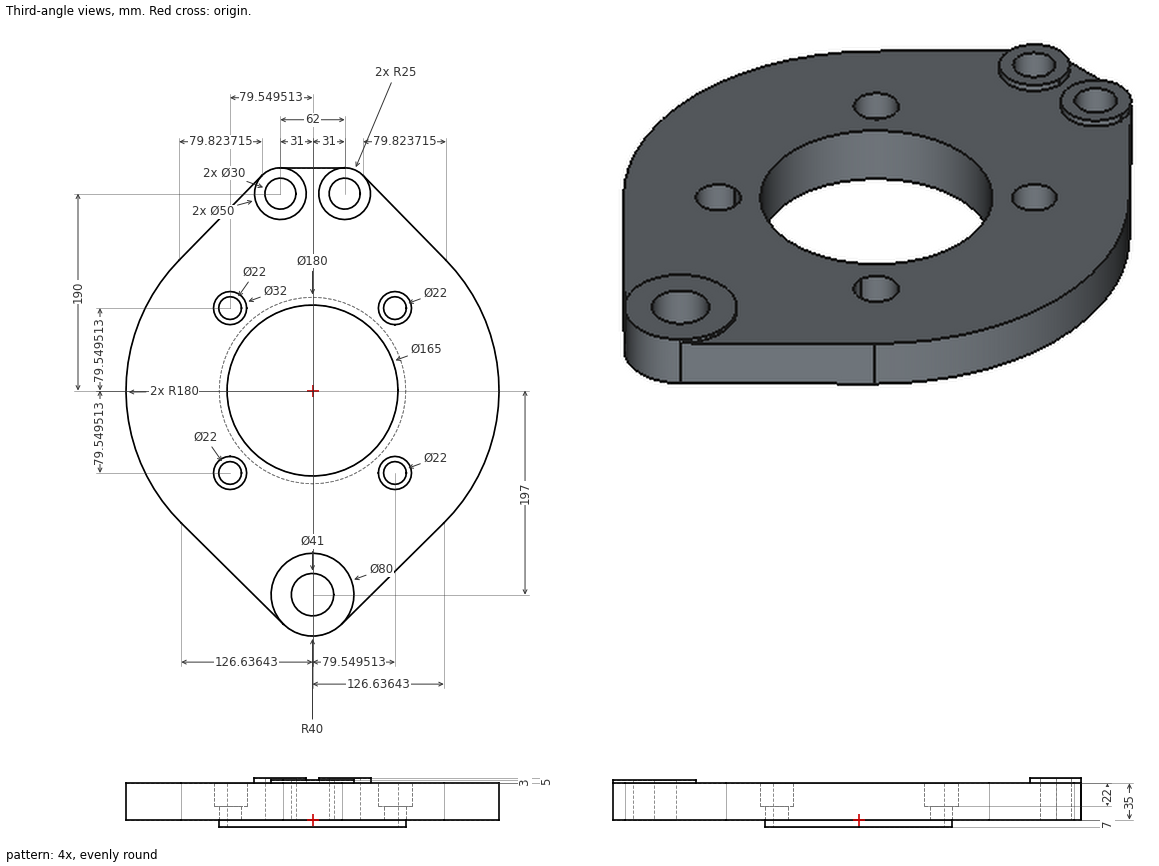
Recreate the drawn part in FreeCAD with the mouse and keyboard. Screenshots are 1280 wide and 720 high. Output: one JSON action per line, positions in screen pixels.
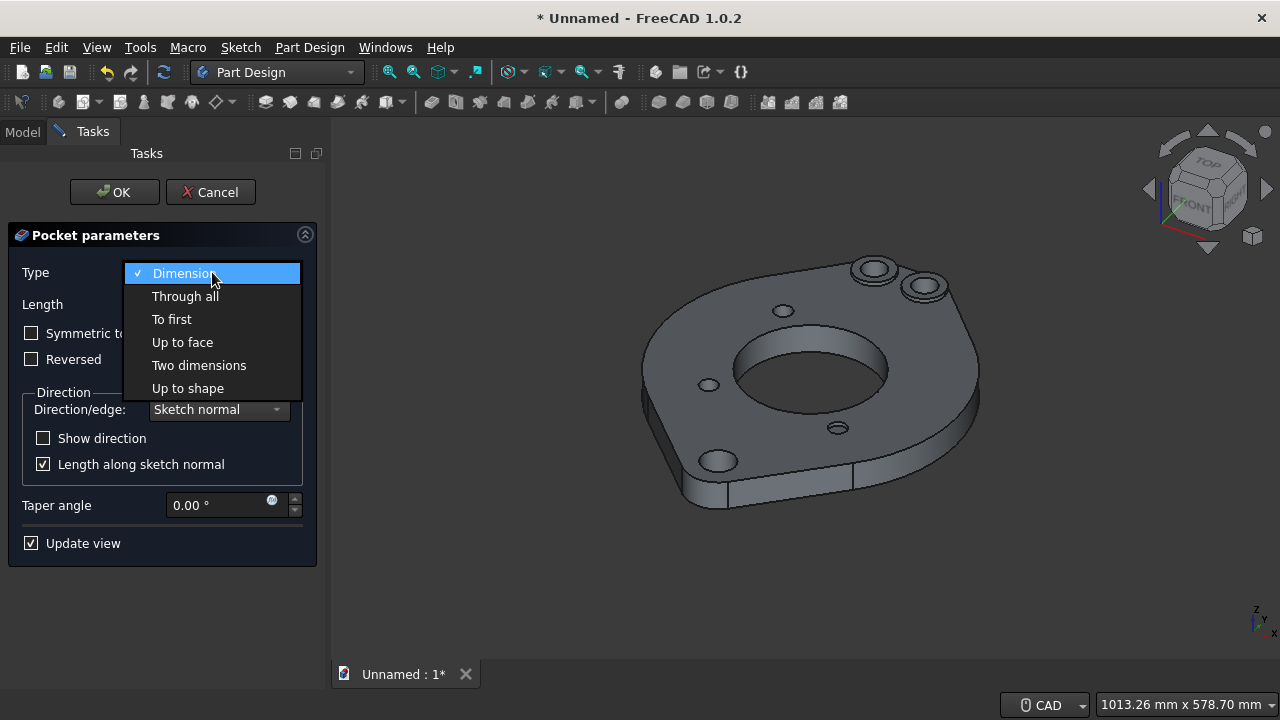
{"action": "left_click", "coordinate": [212, 320]}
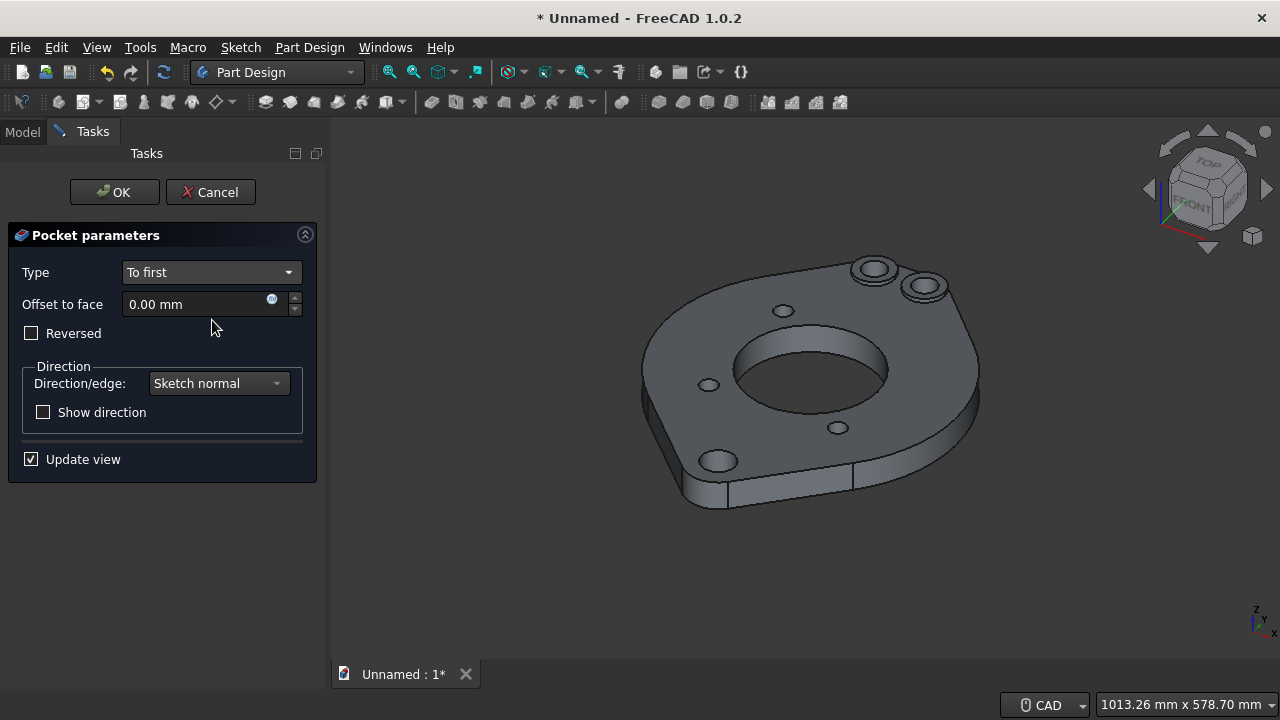
{"action": "left_click", "coordinate": [115, 192]}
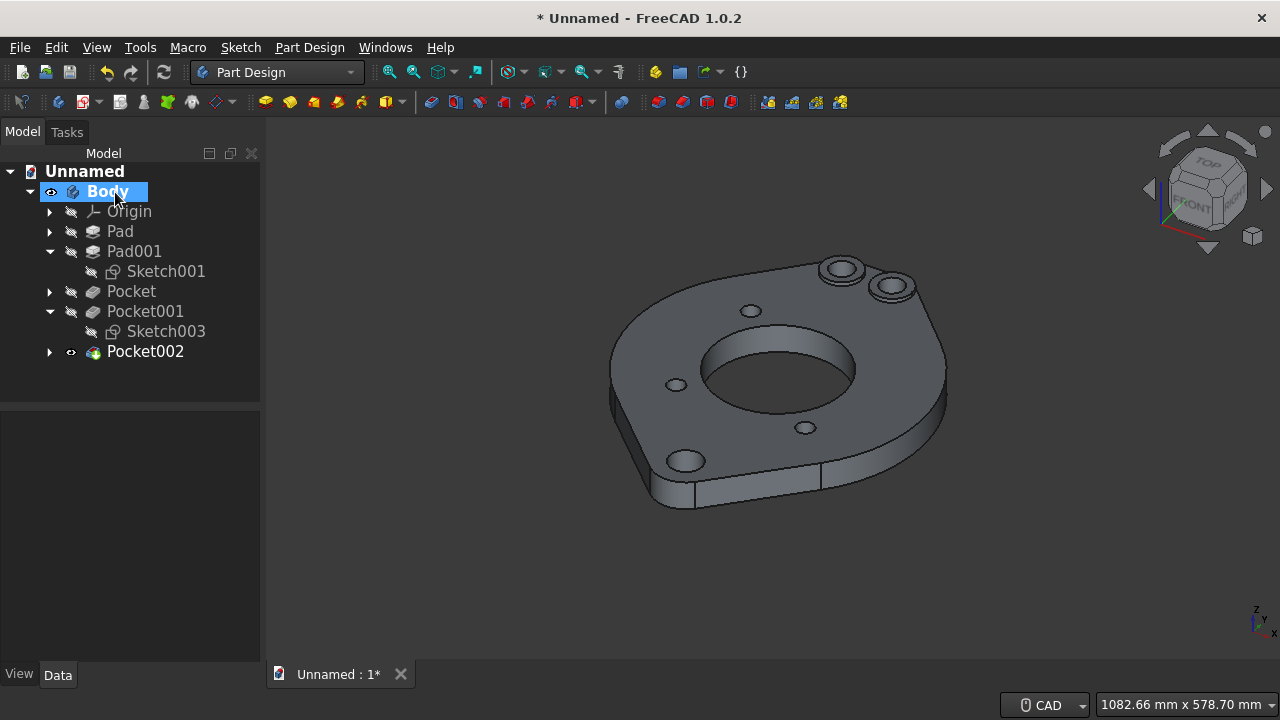
{"action": "left_click", "coordinate": [875, 327]}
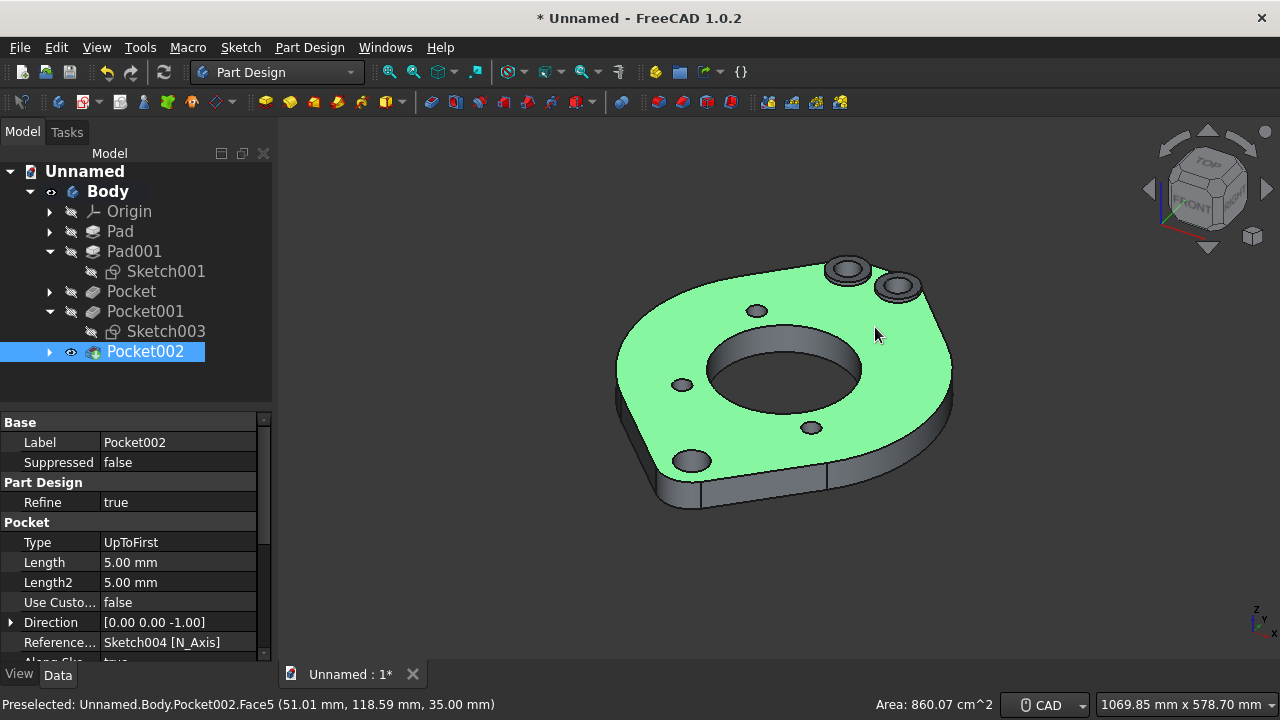
{"action": "left_click", "coordinate": [84, 102]}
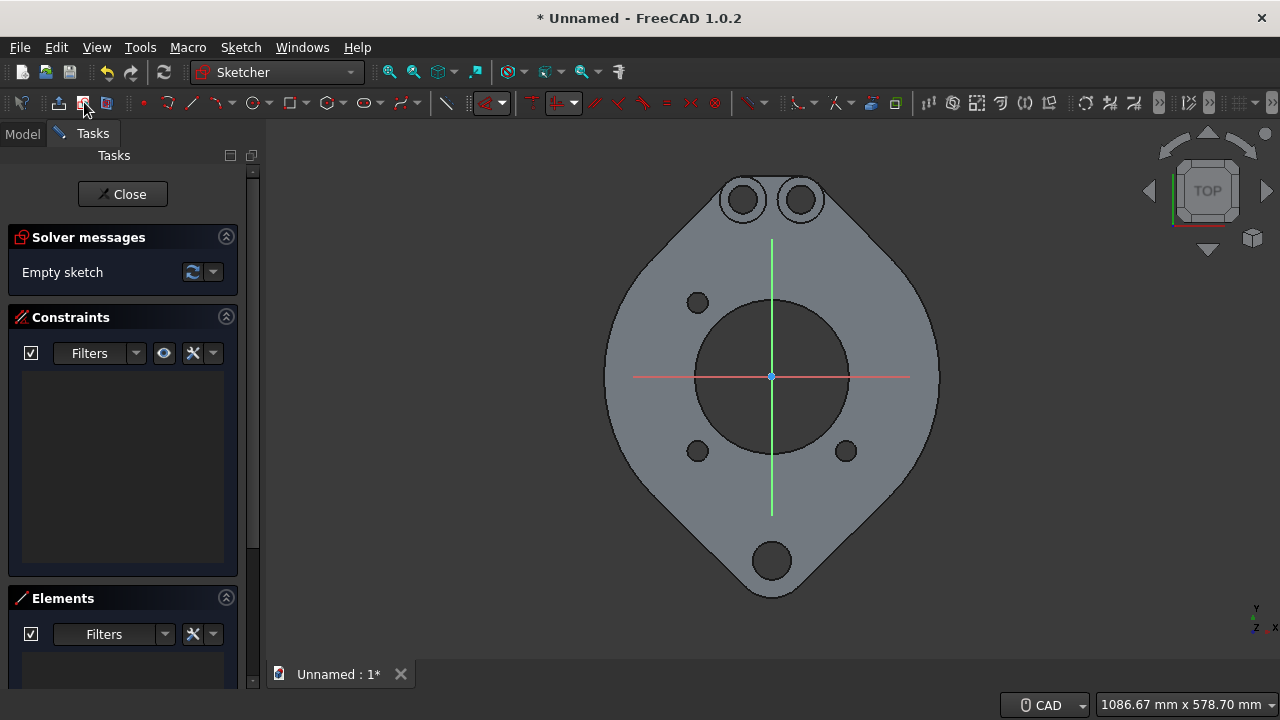
{"action": "scroll", "coordinate": [855, 297], "scroll_direction": "up", "scroll_amount": 14}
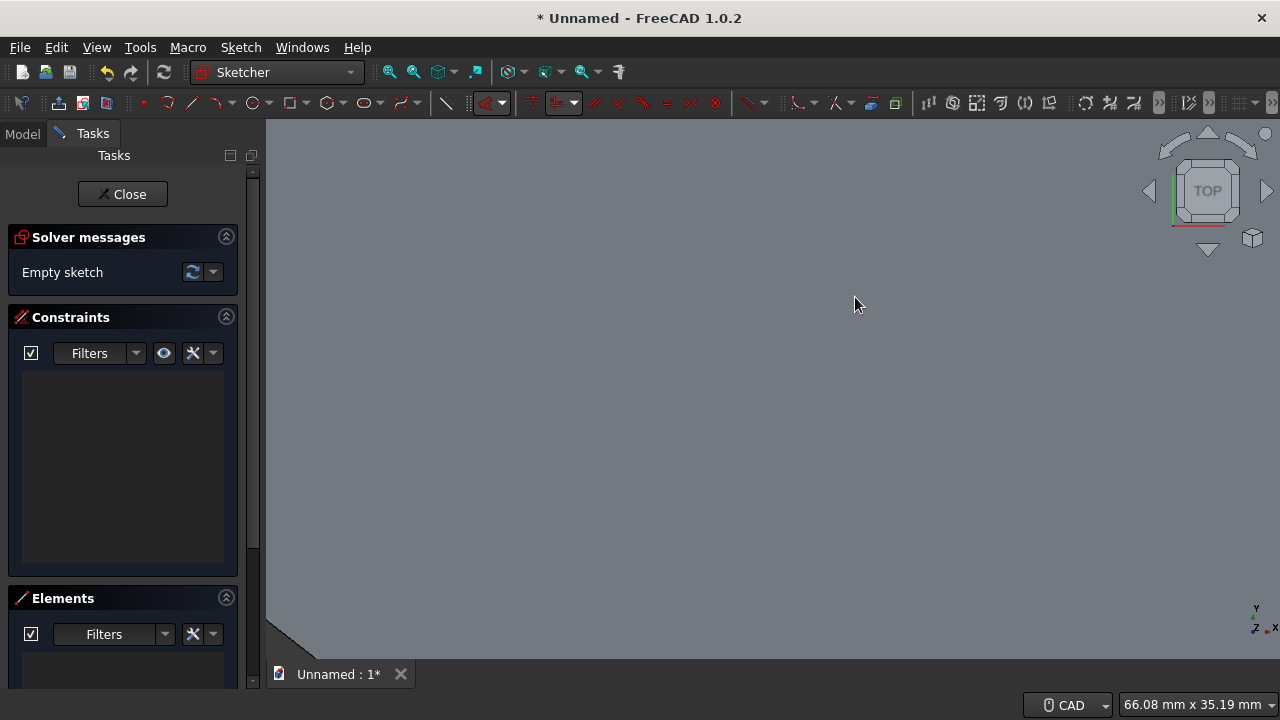
{"action": "key", "text": "g c"}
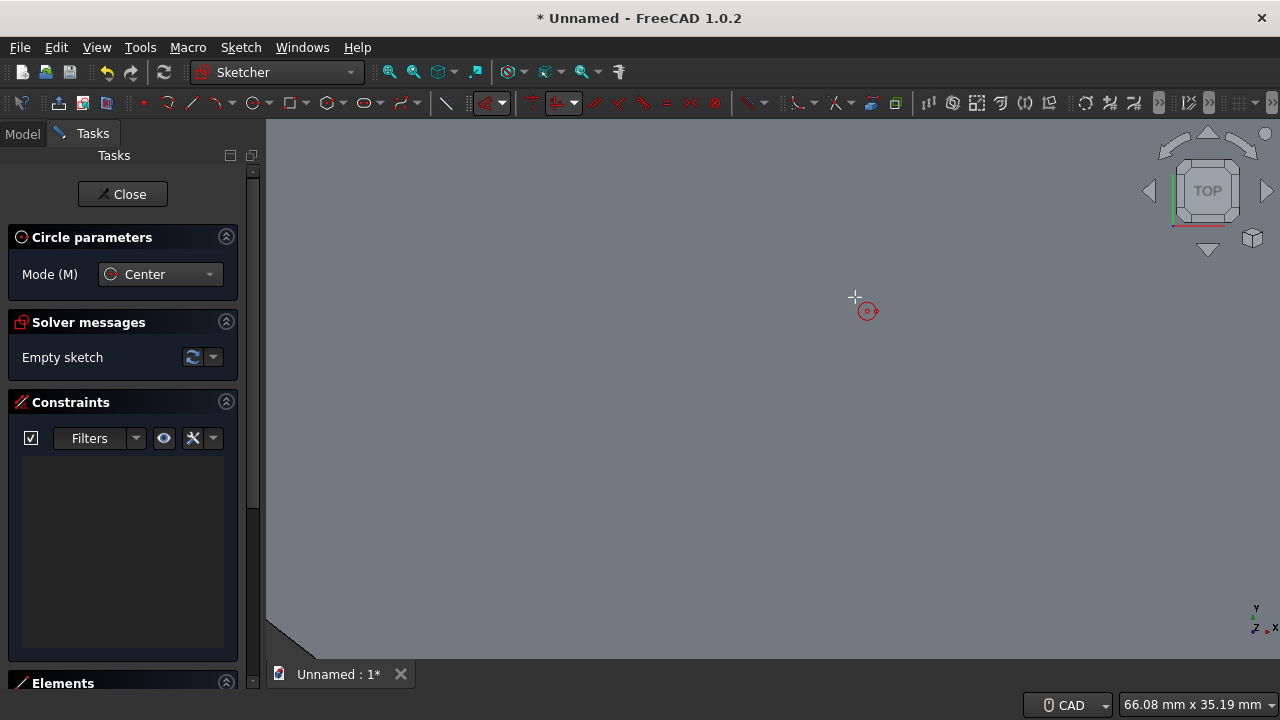
{"action": "left_click", "coordinate": [700, 386]}
{"action": "left_click", "coordinate": [820, 267]}
{"action": "key", "text": "Escape"}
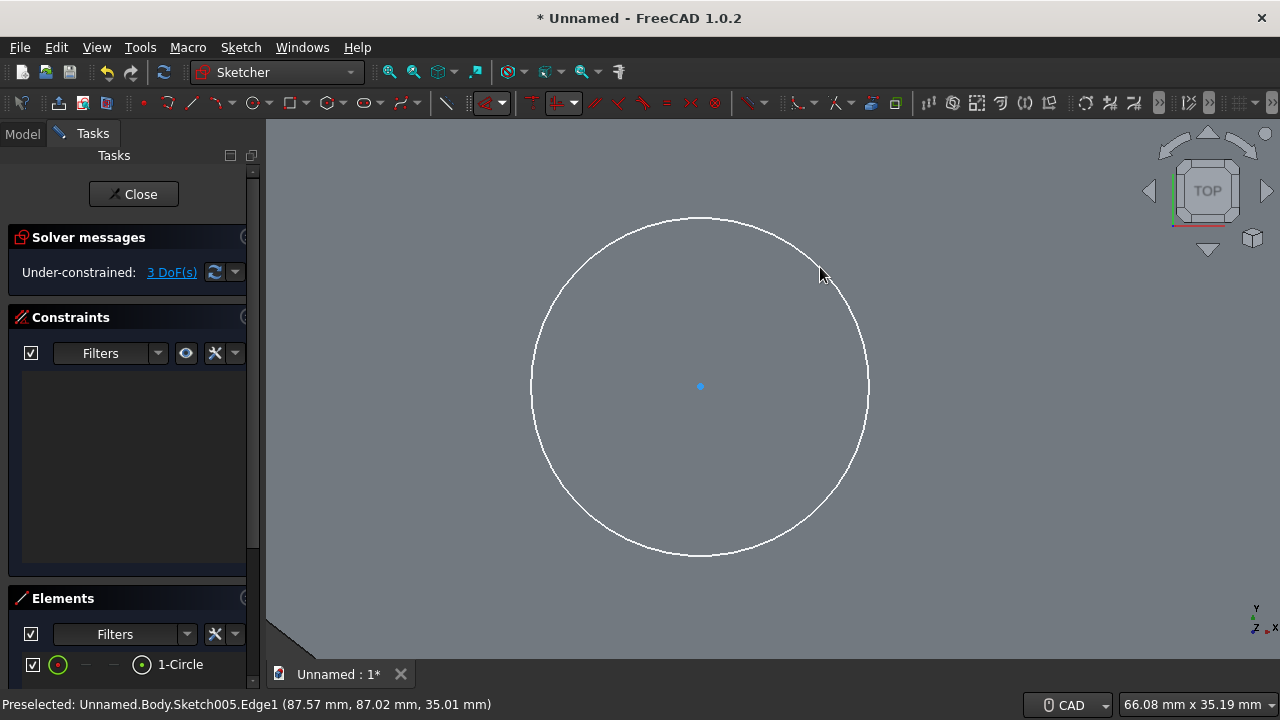
{"action": "left_click", "coordinate": [819, 267]}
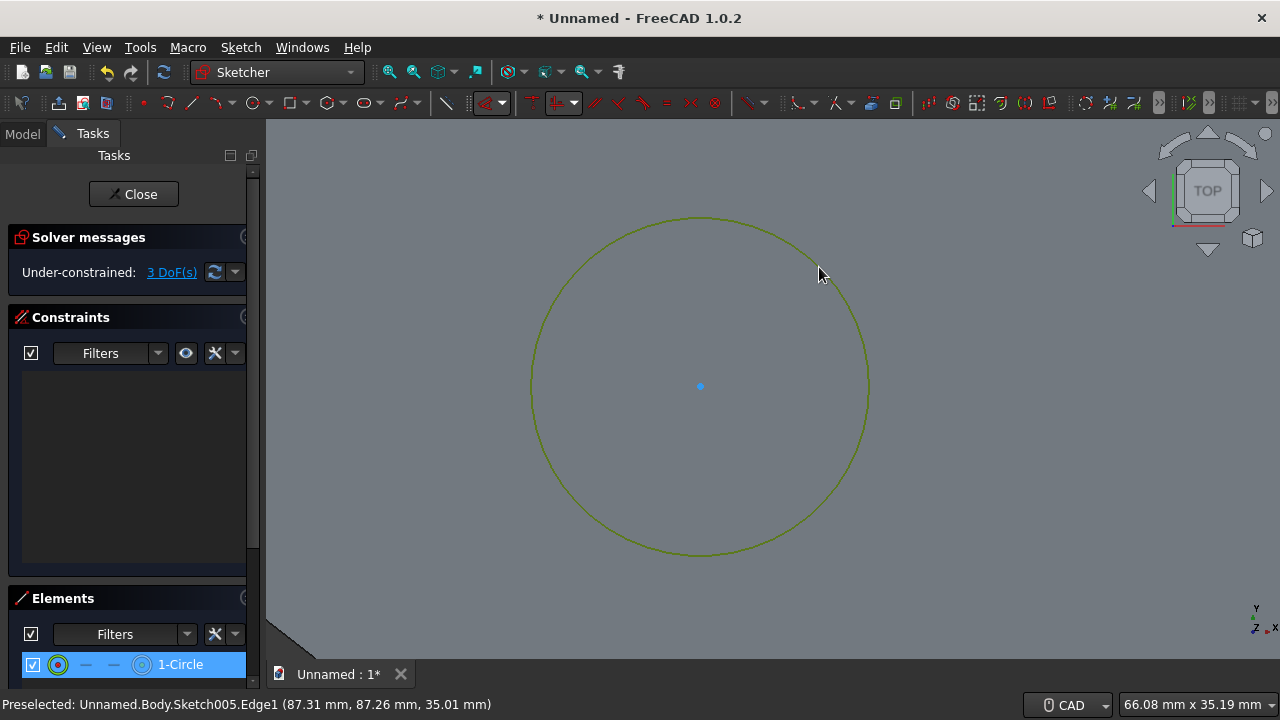
{"action": "left_click", "coordinate": [504, 104]}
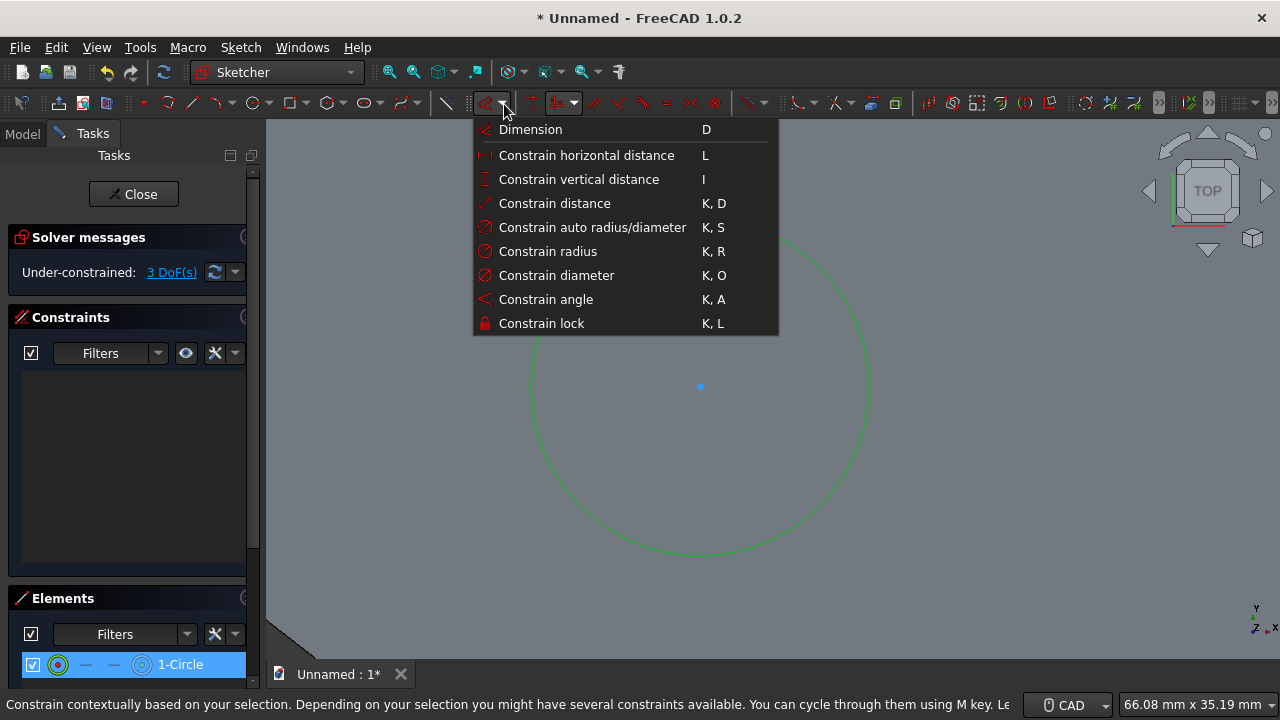
{"action": "left_click", "coordinate": [626, 275]}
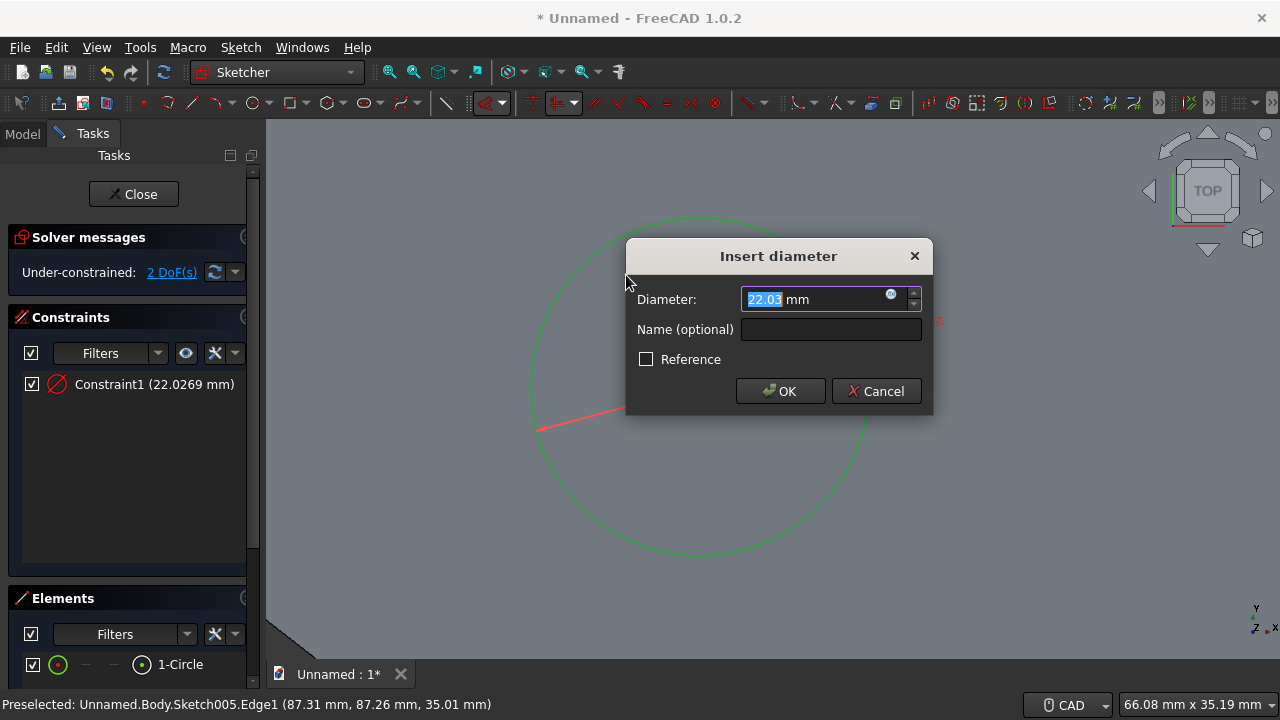
{"action": "type", "text": "22"}
{"action": "key", "text": "Return"}